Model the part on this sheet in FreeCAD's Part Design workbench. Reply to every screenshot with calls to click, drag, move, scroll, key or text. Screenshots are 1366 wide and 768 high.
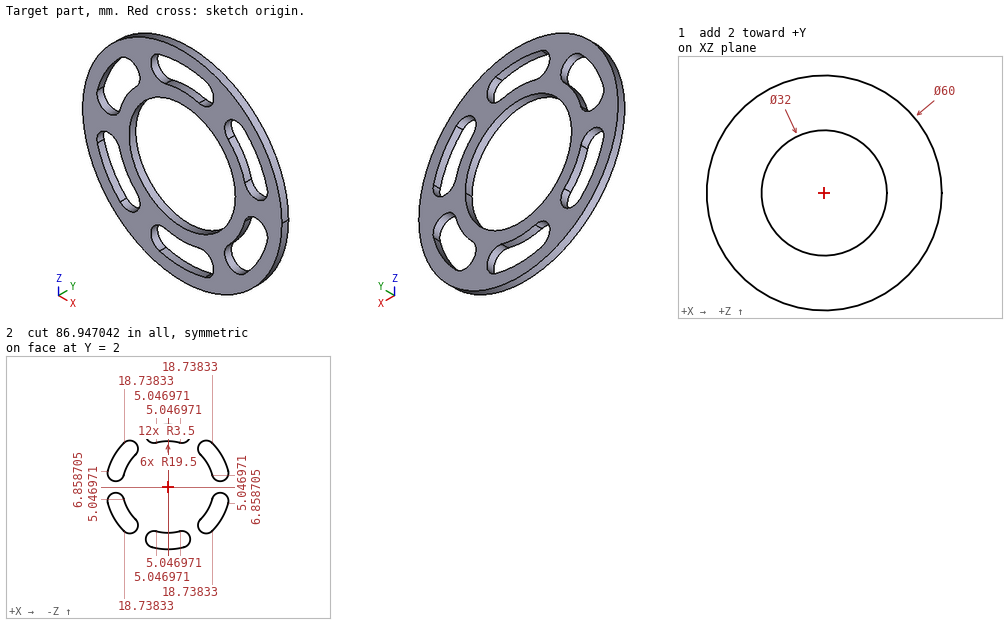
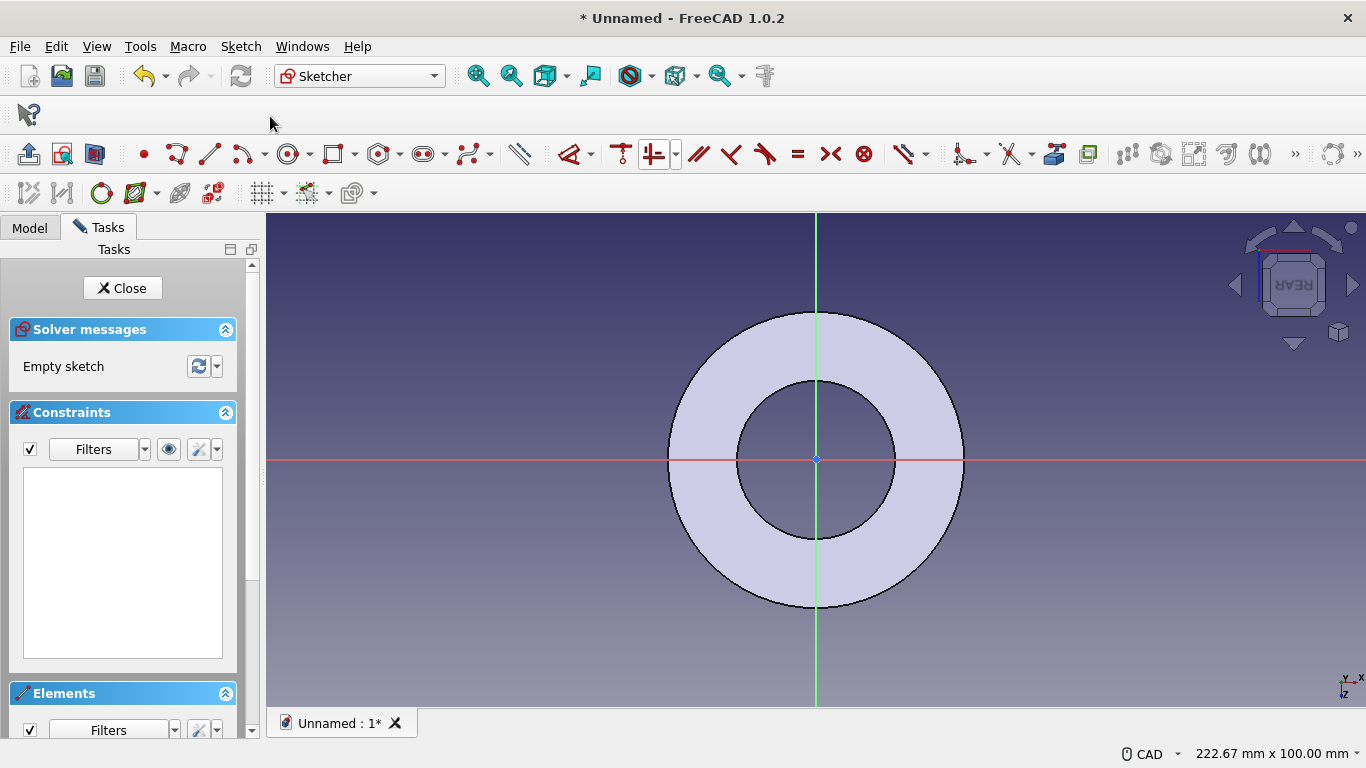
key(g)
key(3)
key(a)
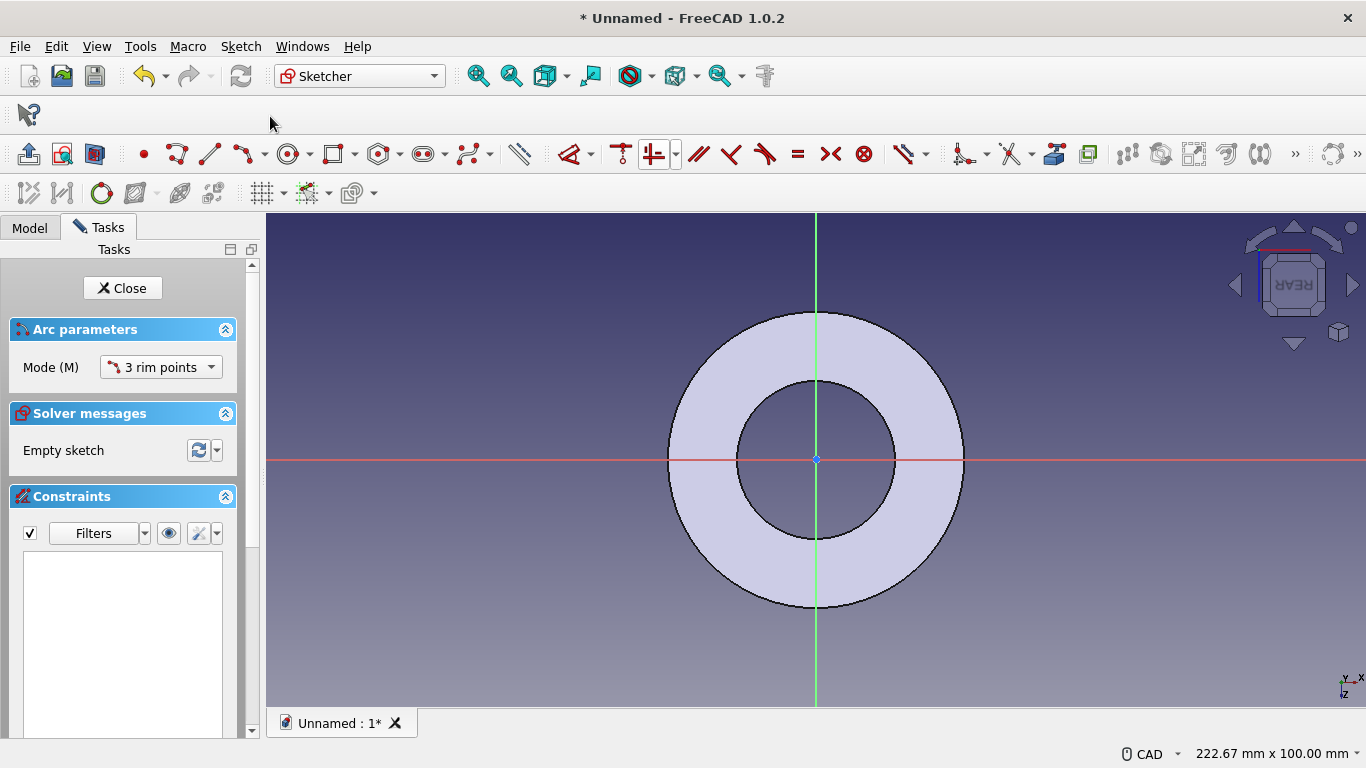
click(791, 367)
click(841, 367)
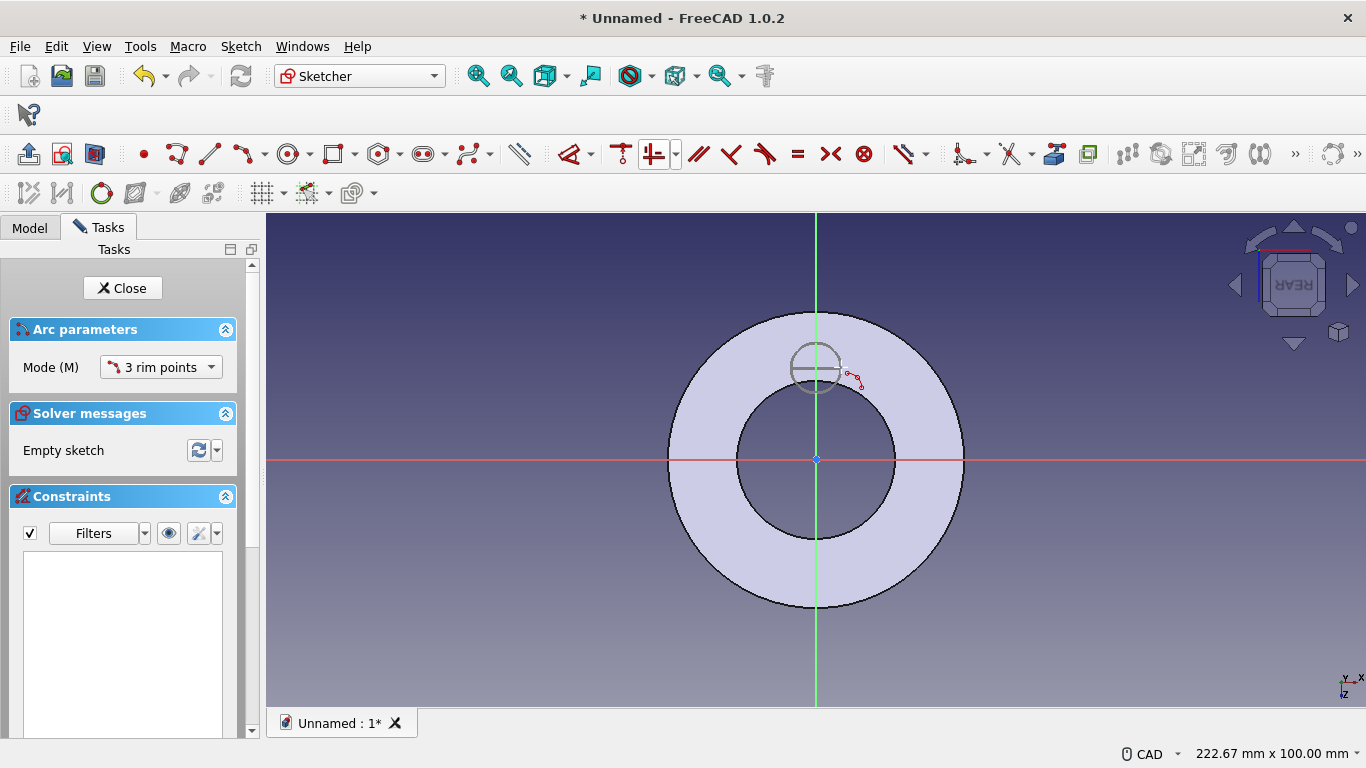
scroll(821, 364, up, 9)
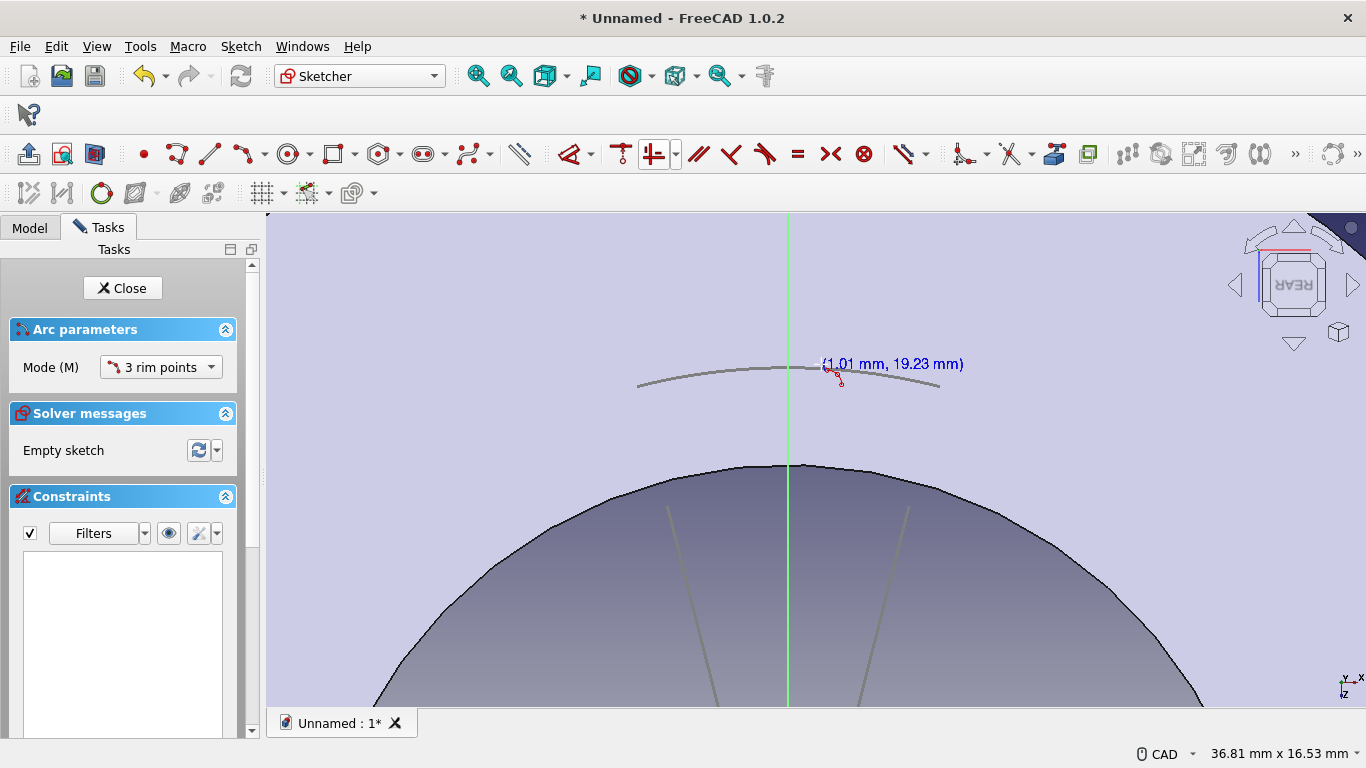
click(819, 361)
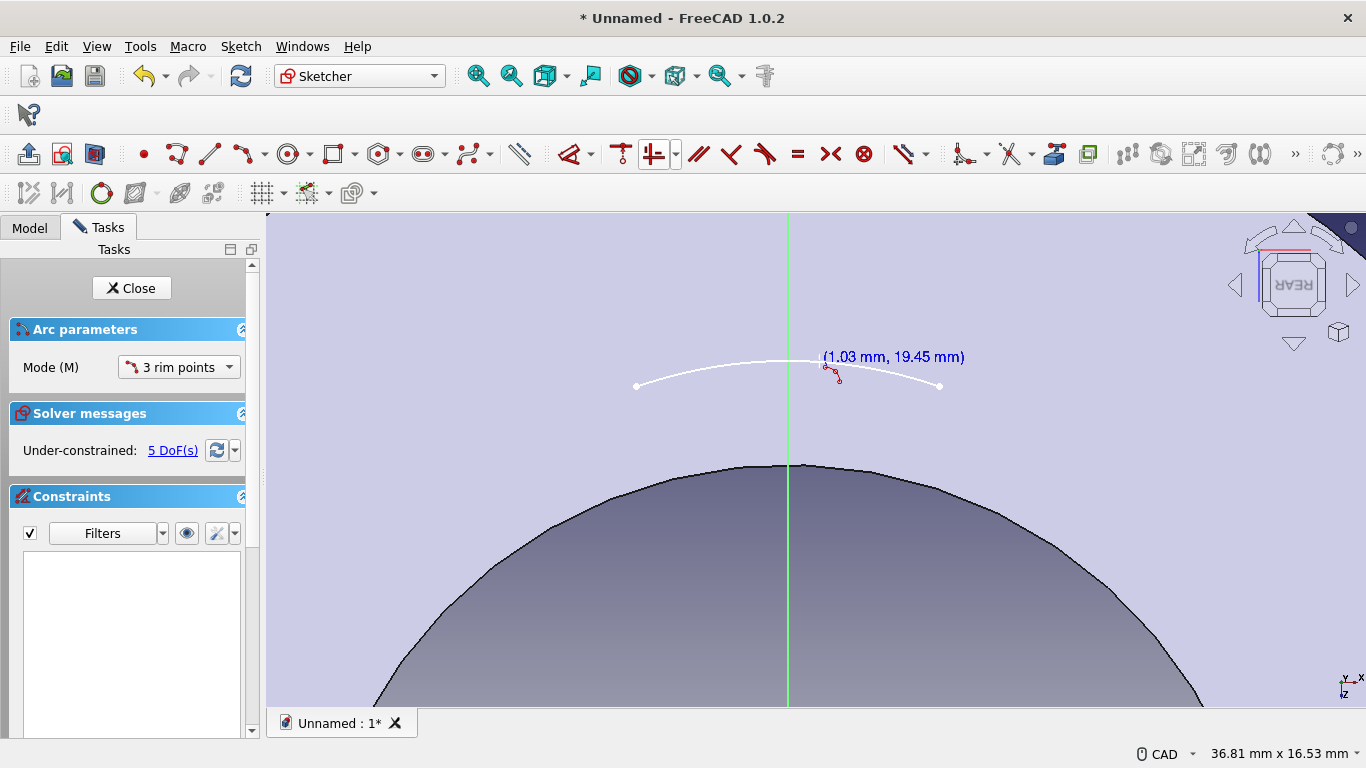
scroll(737, 338, down, 8)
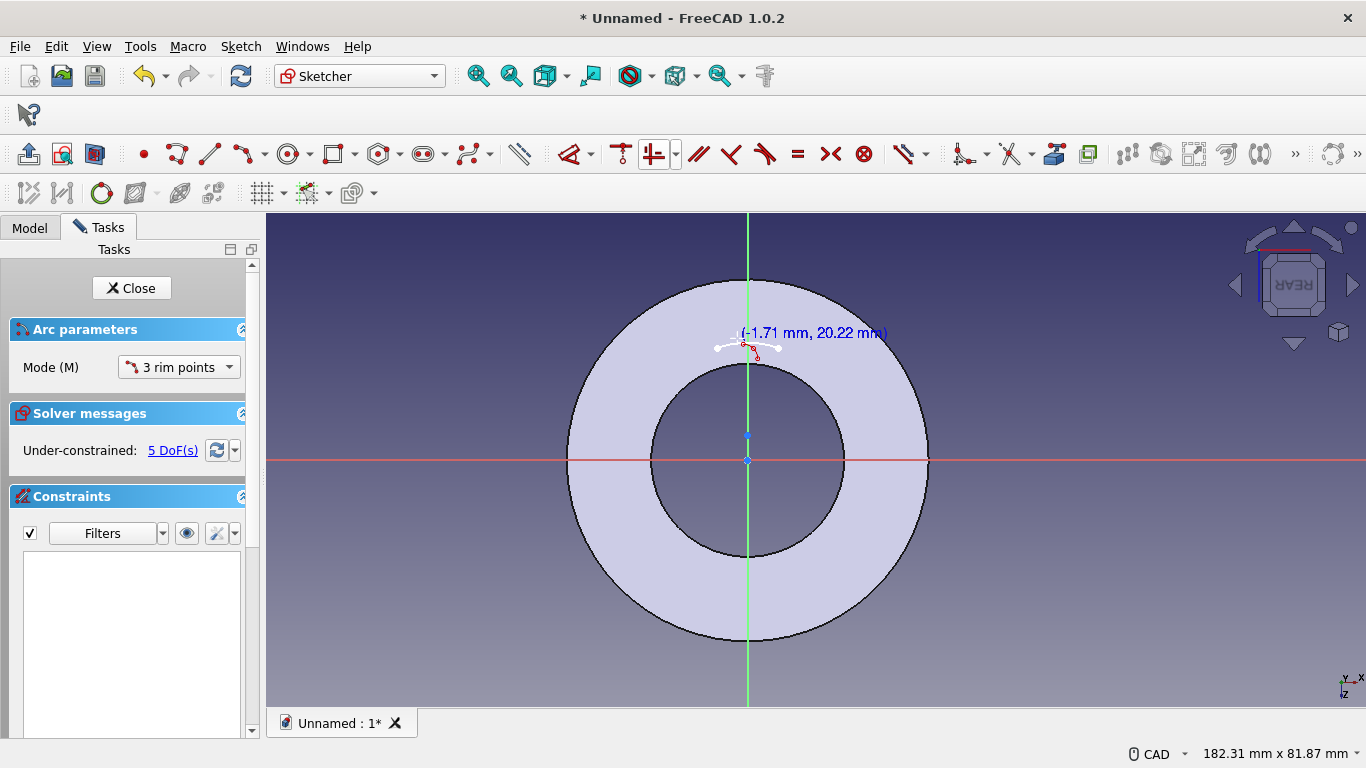
click(778, 348)
click(789, 306)
click(804, 332)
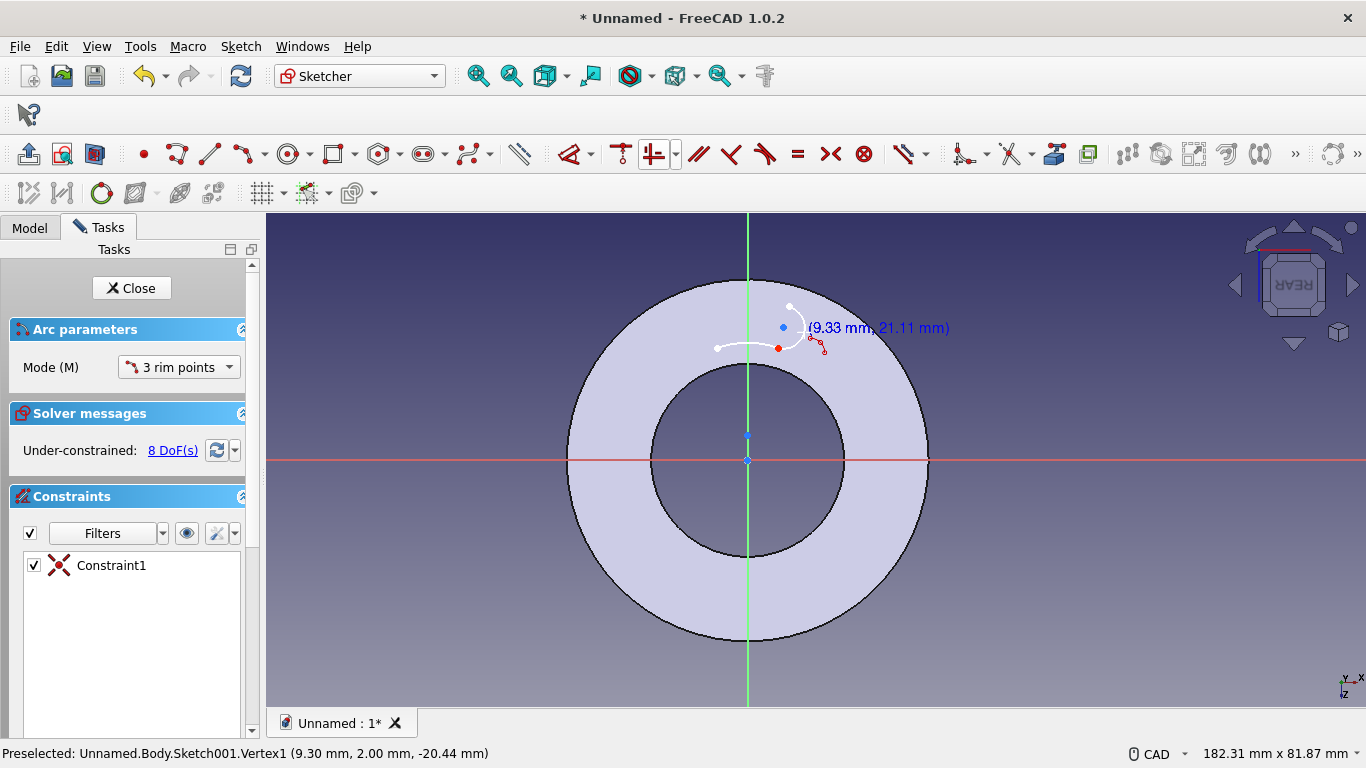
click(789, 307)
click(706, 306)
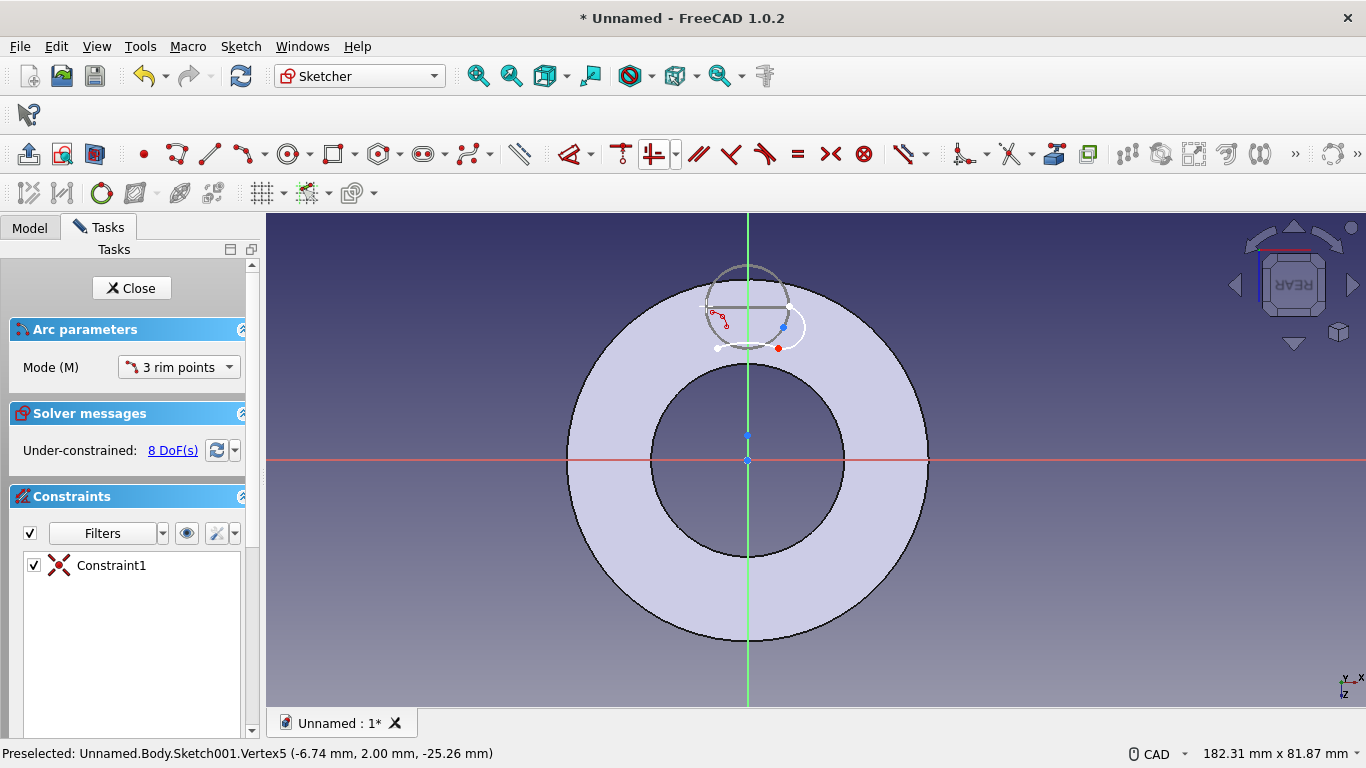
scroll(756, 301, up, 6)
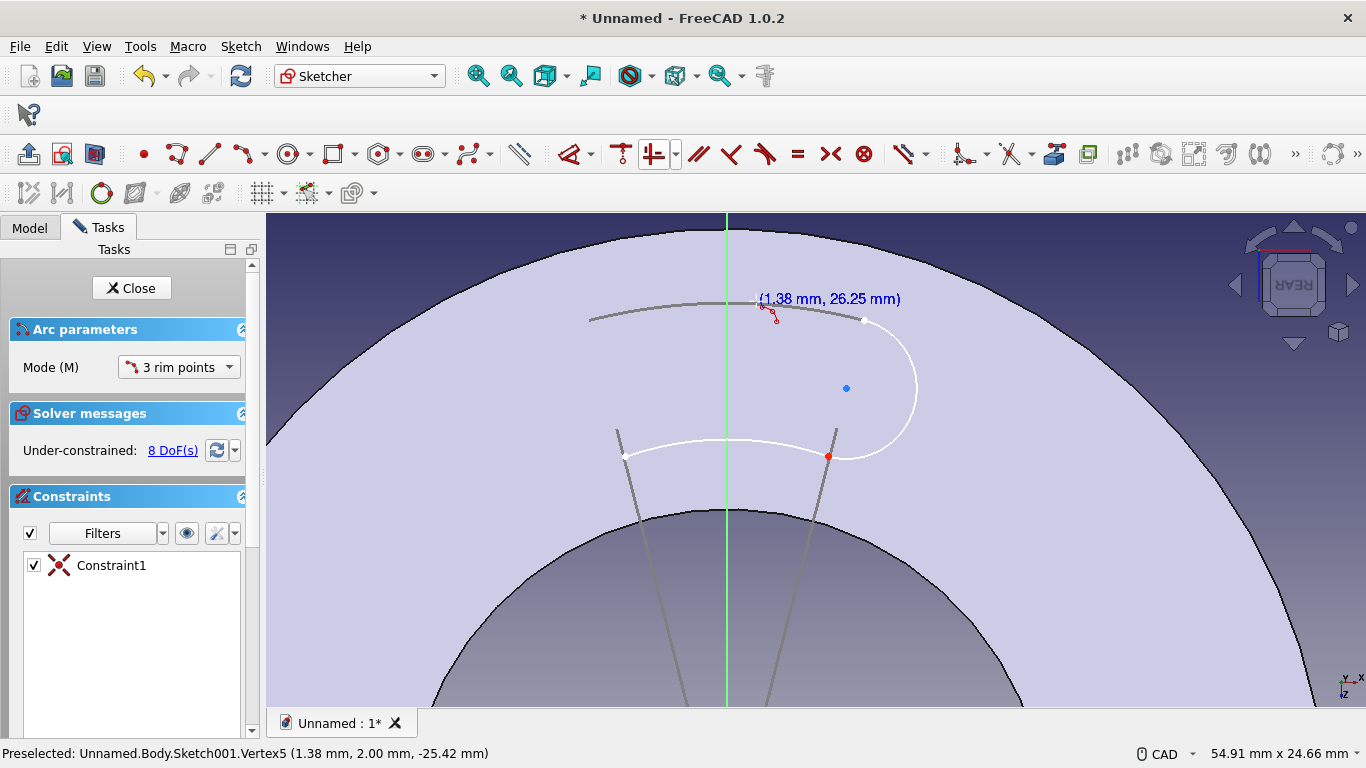
click(755, 300)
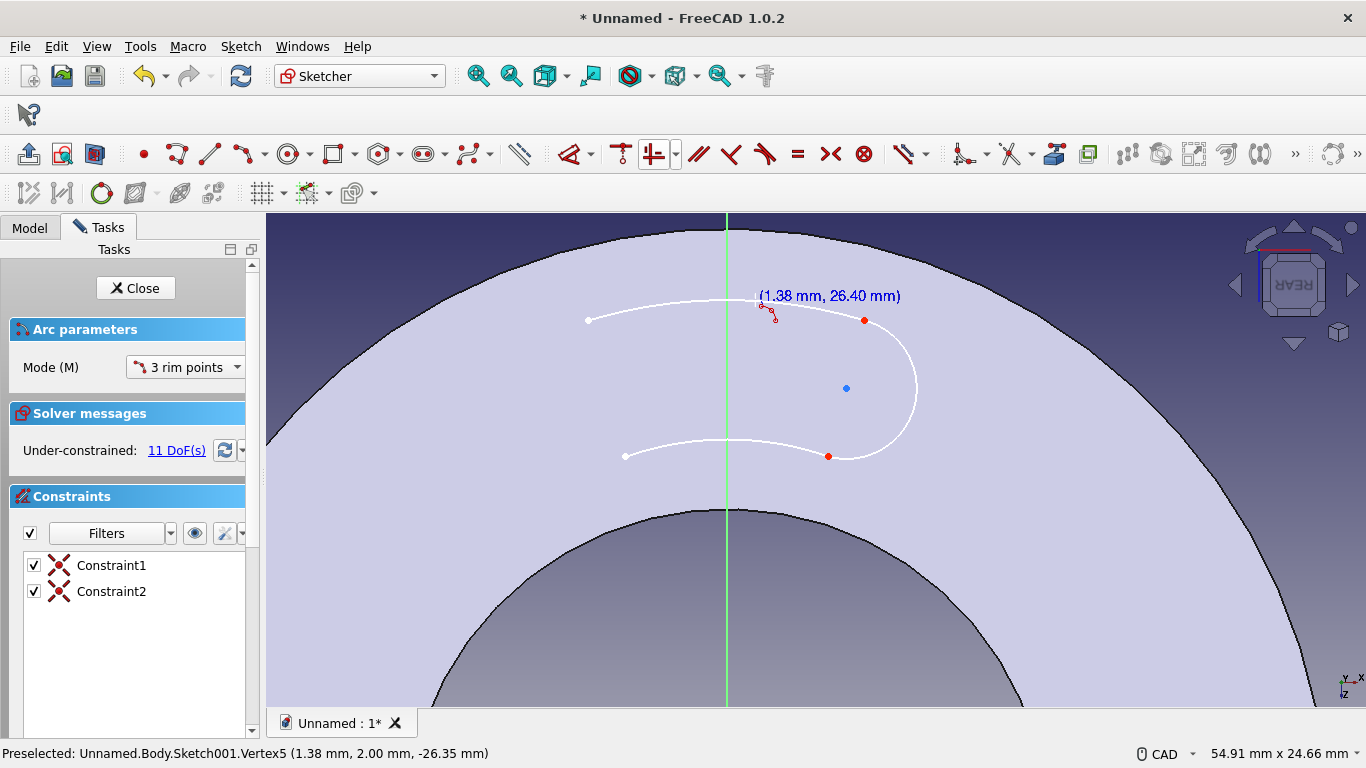
scroll(756, 301, down, 6)